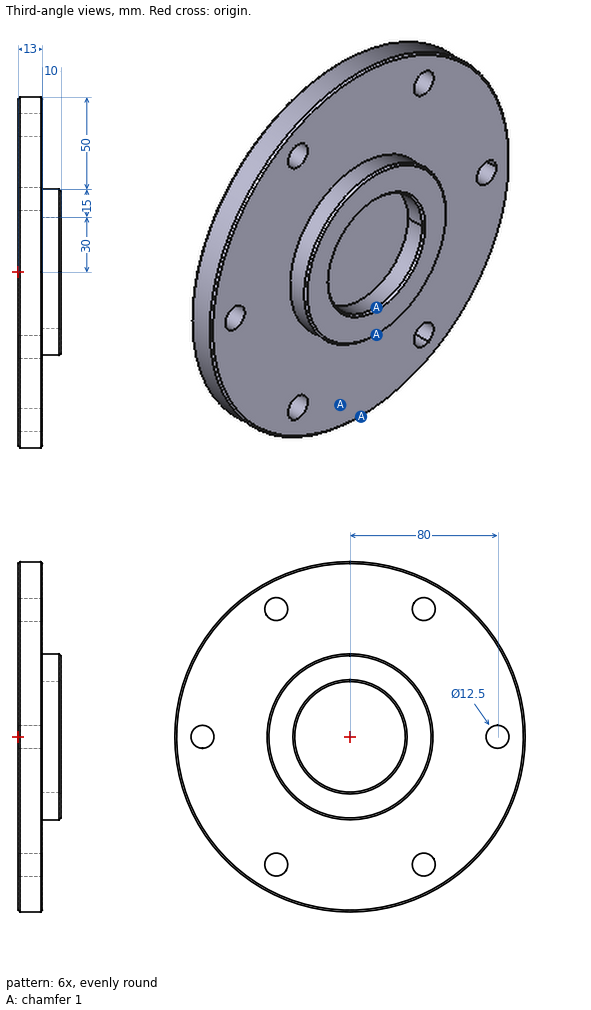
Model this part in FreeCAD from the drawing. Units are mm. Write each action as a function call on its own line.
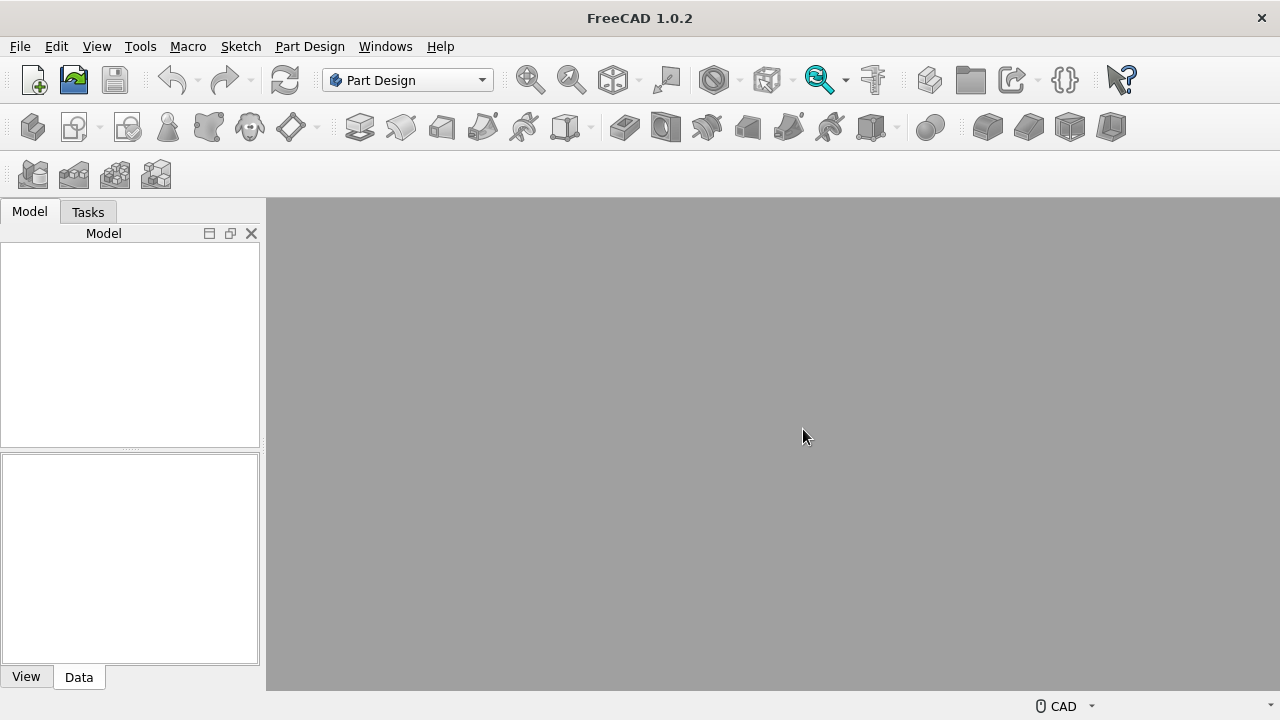
click(33, 80)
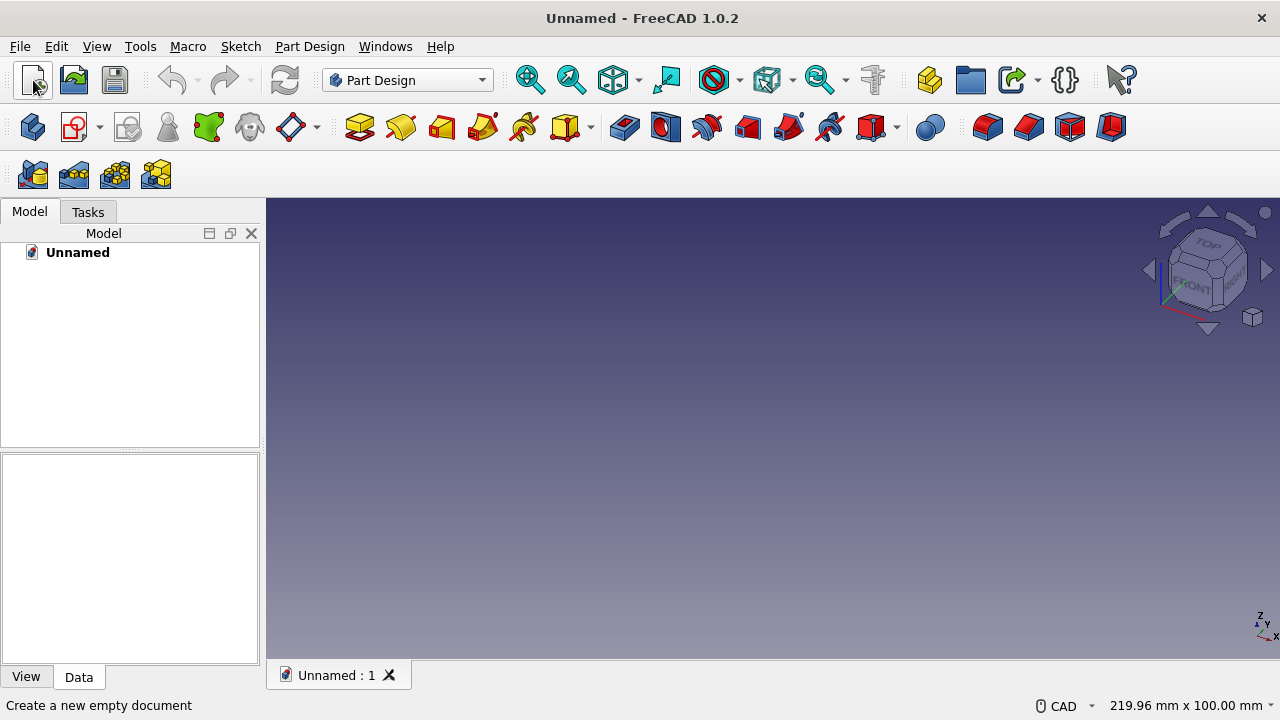
click(74, 128)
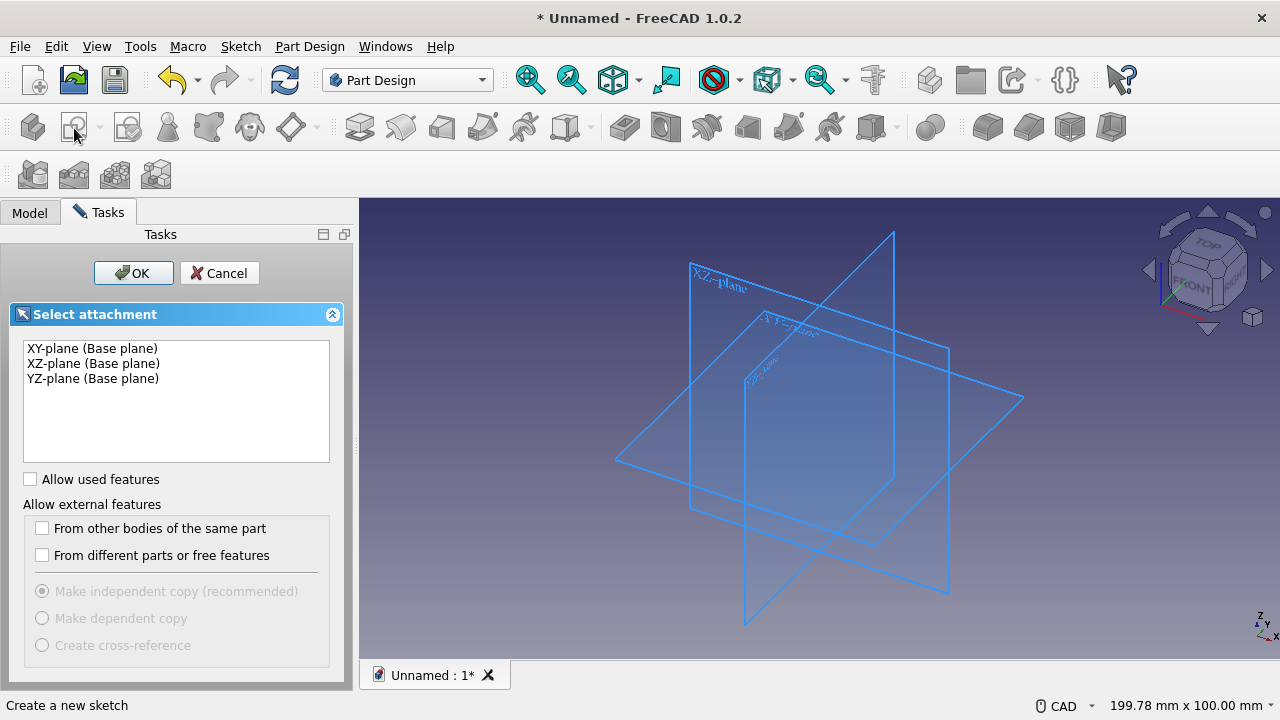
click(84, 348)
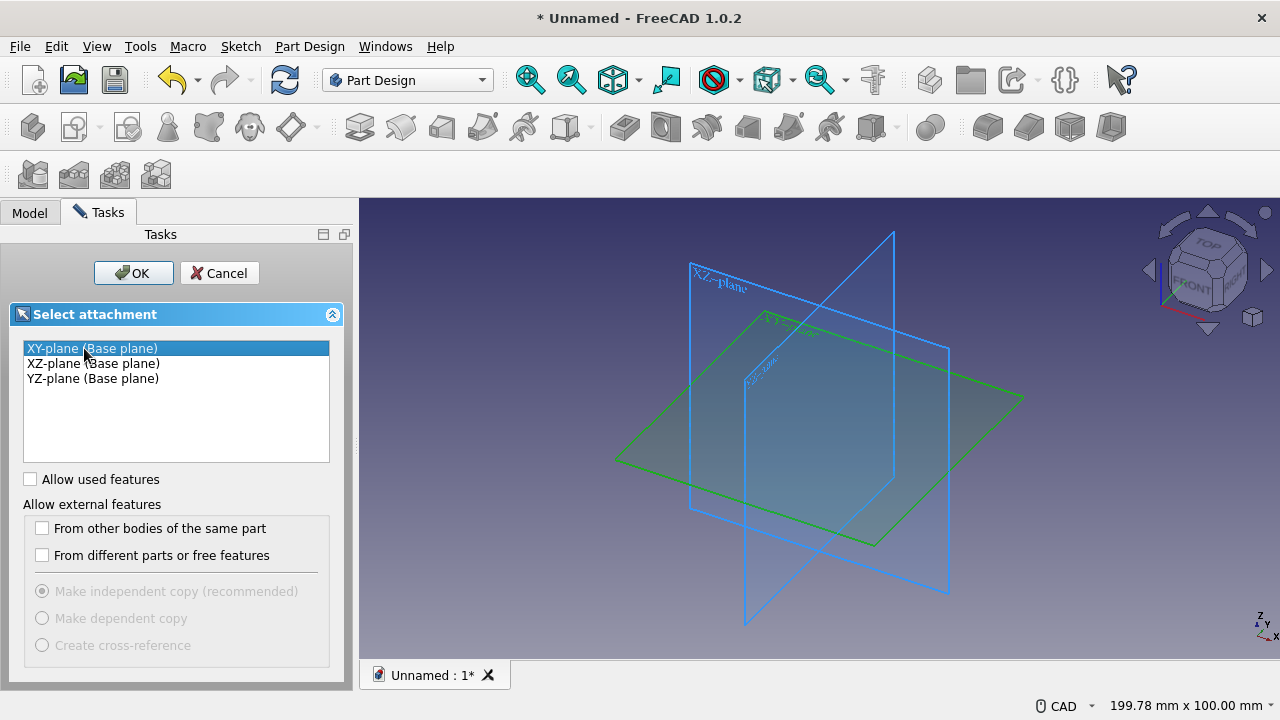
click(134, 273)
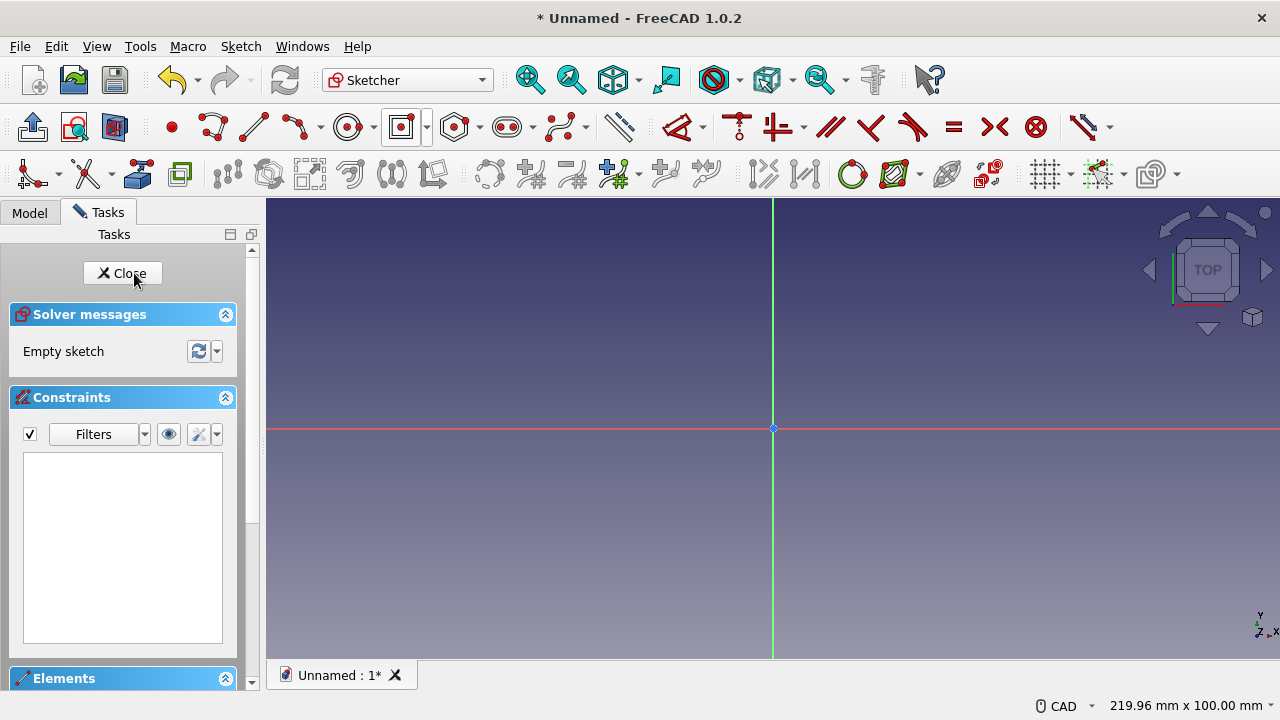
scroll(557, 631, down, 3)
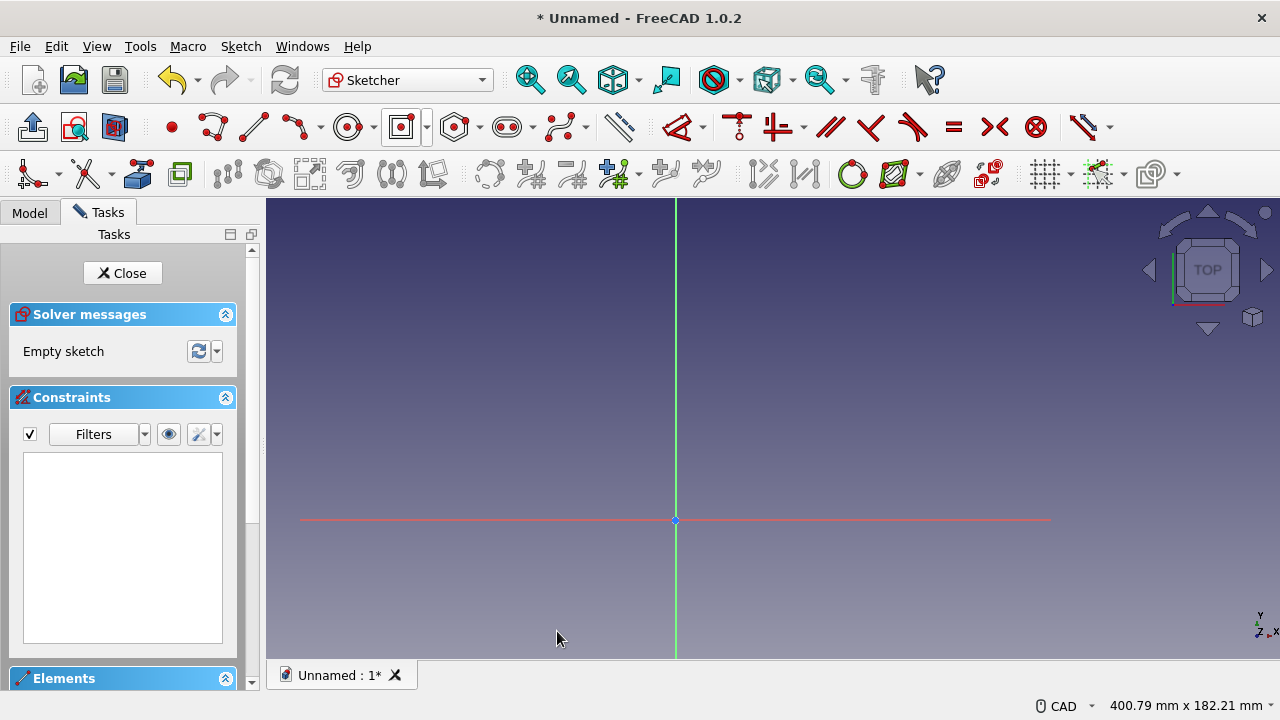
key(g)
key(m)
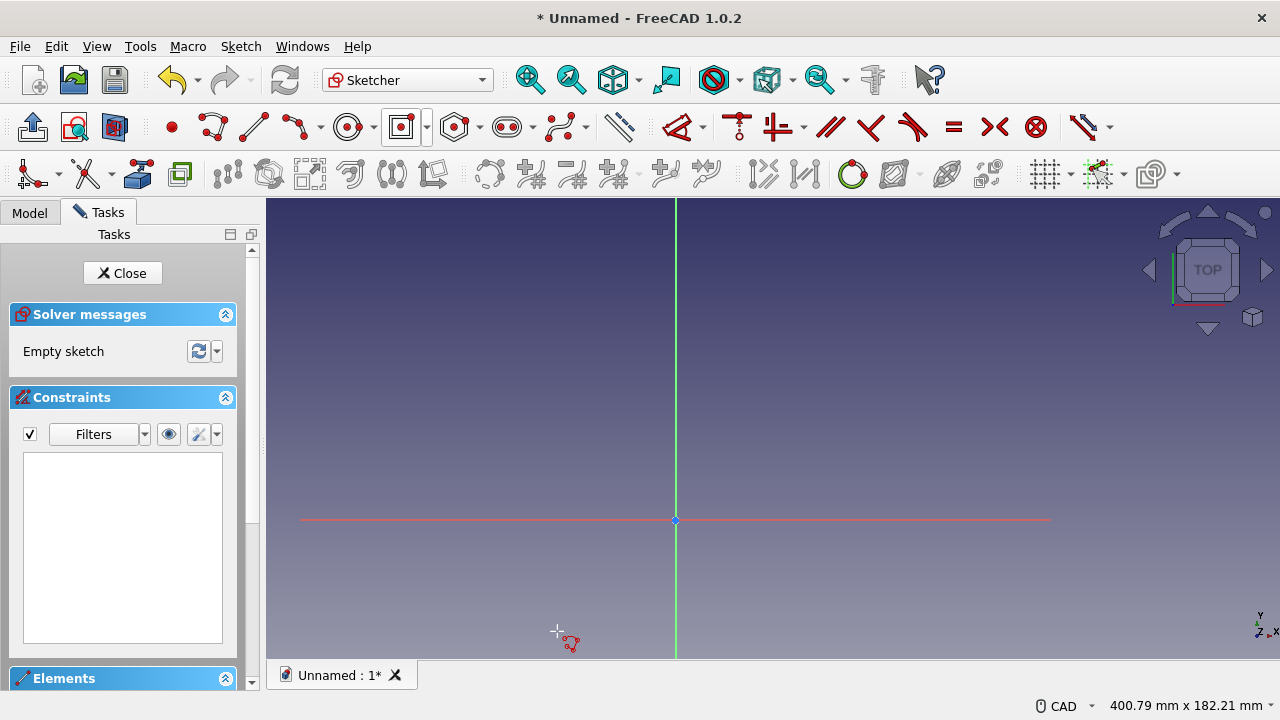
click(676, 520)
click(709, 511)
click(709, 444)
click(734, 444)
click(734, 406)
click(709, 406)
click(709, 280)
click(685, 280)
click(676, 520)
key(Escape)
key(Escape)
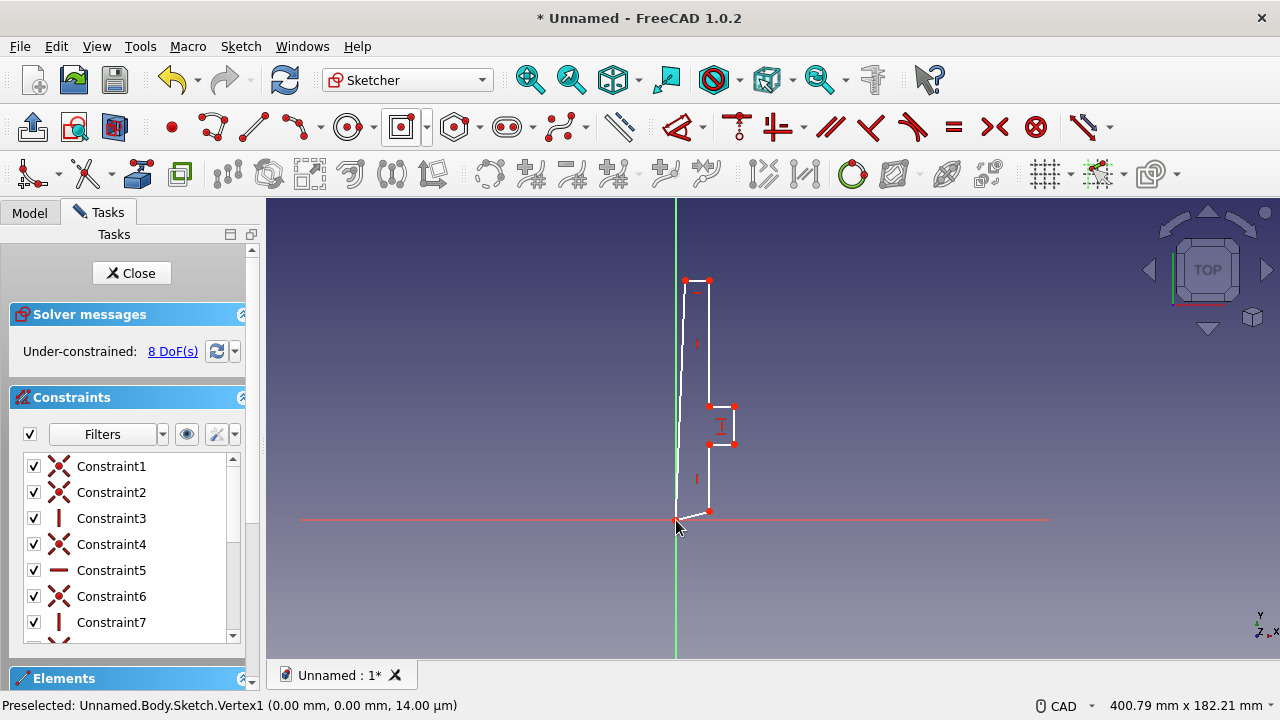
scroll(686, 518, up, 2)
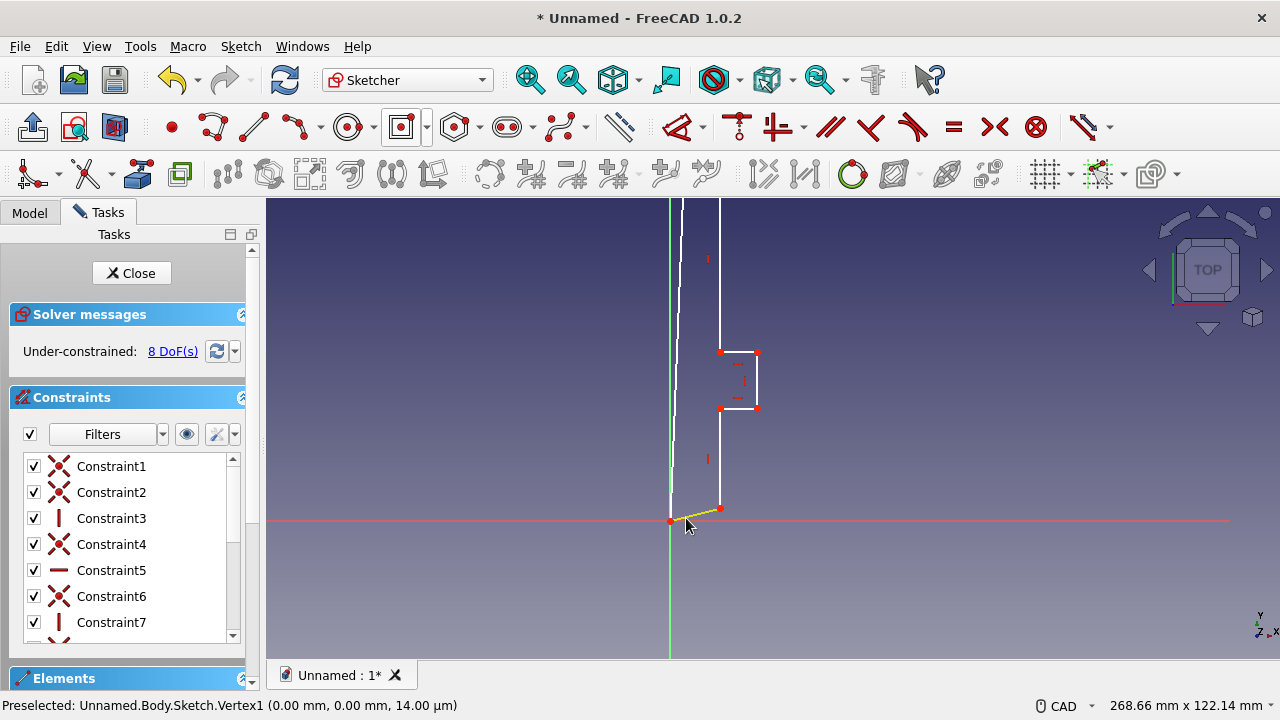
click(685, 517)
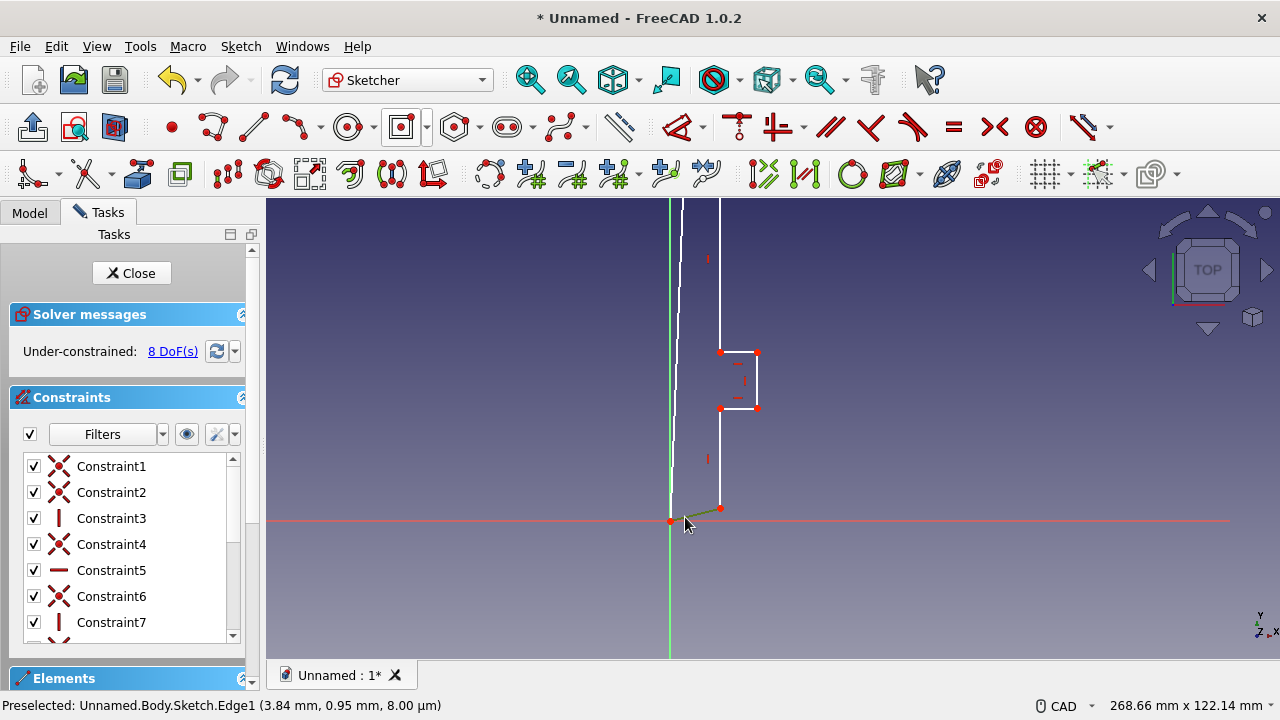
key(h)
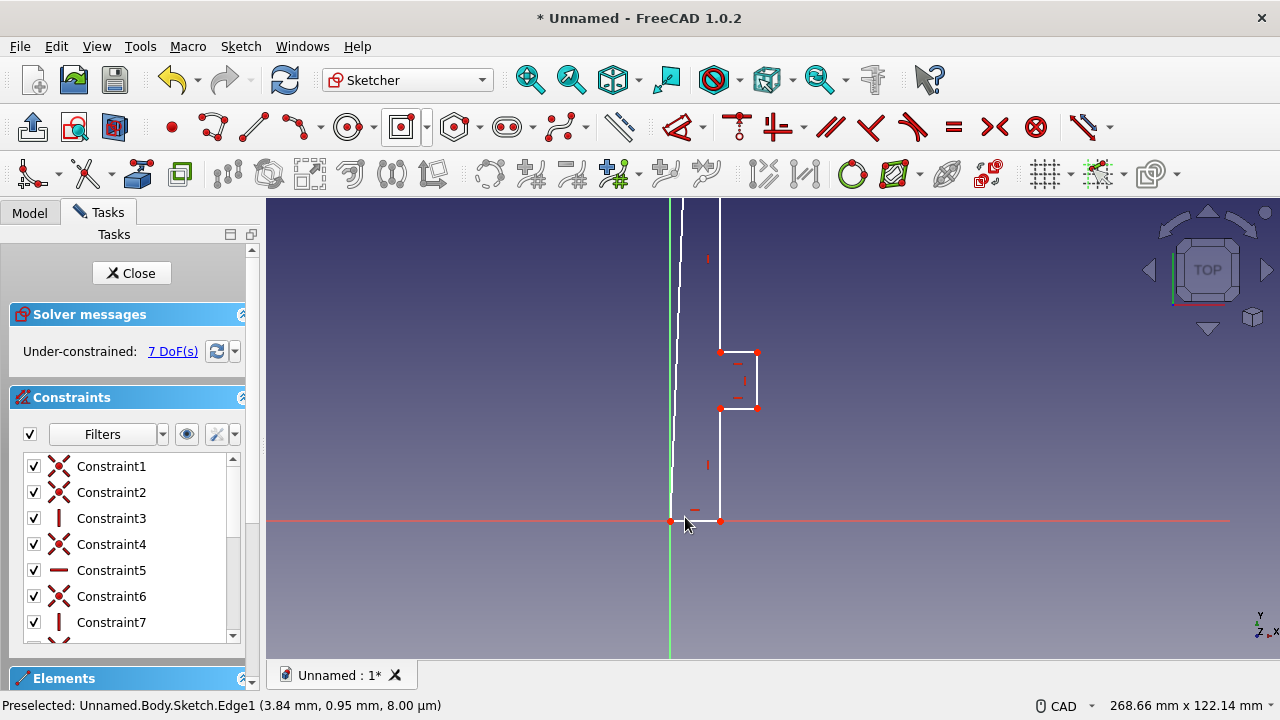
scroll(680, 271, up, 2)